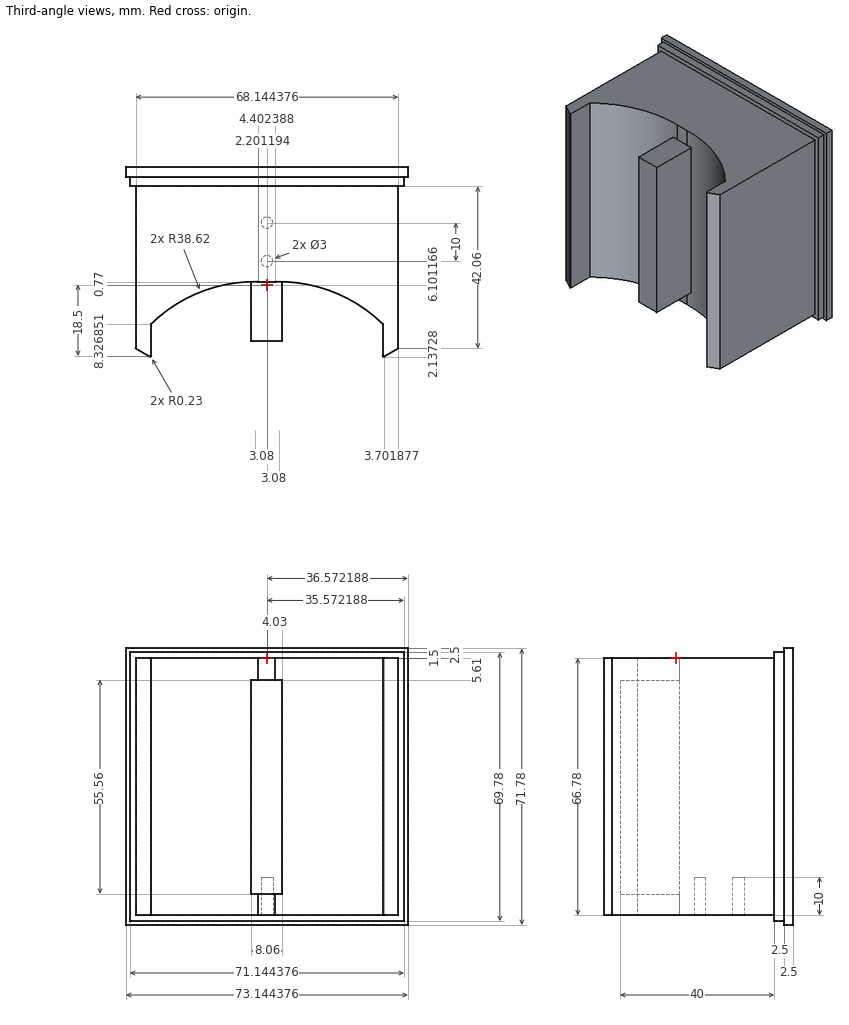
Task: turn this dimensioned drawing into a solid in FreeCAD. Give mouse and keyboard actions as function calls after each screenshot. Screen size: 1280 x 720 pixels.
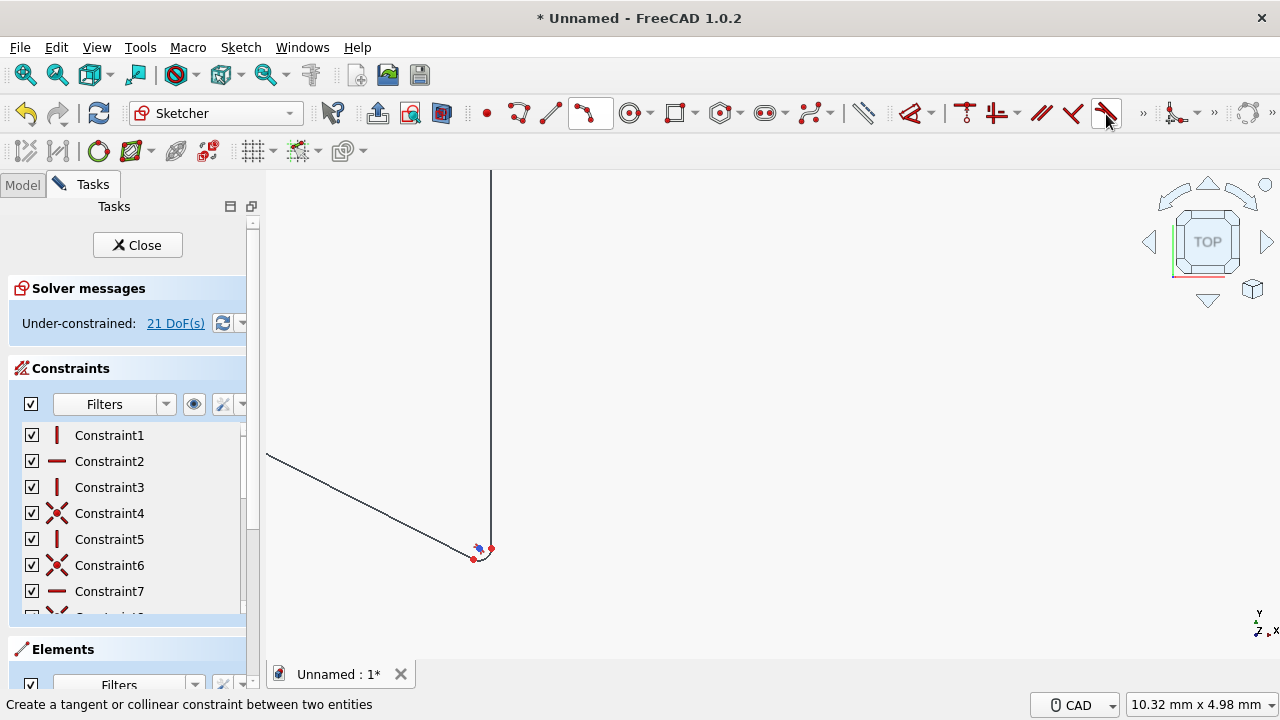
scroll(484, 577, down, 13)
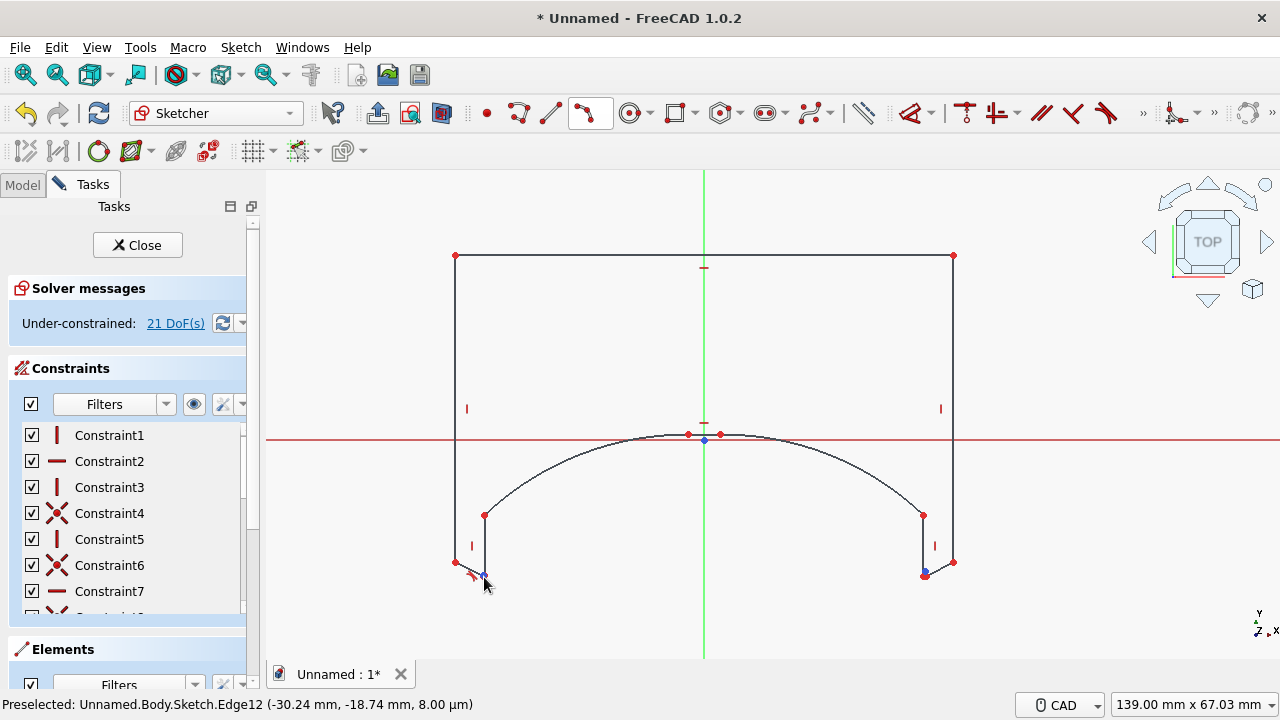
click(923, 534)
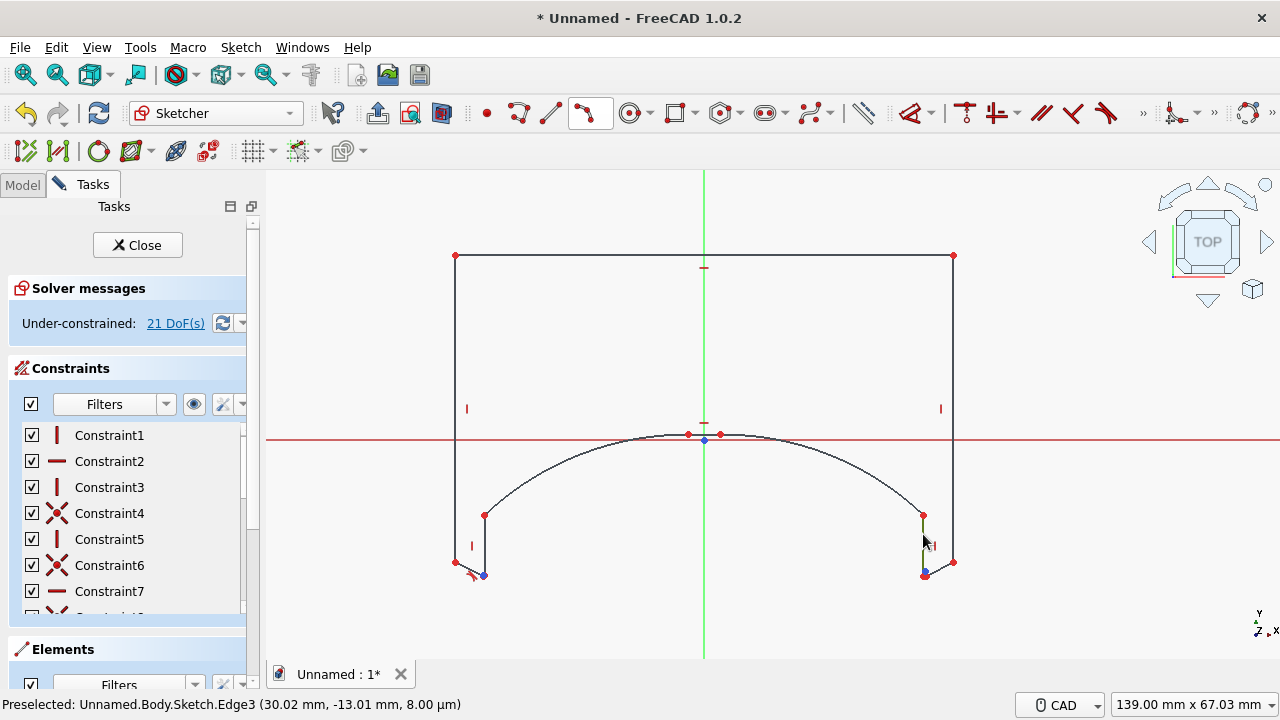
scroll(925, 577, up, 12)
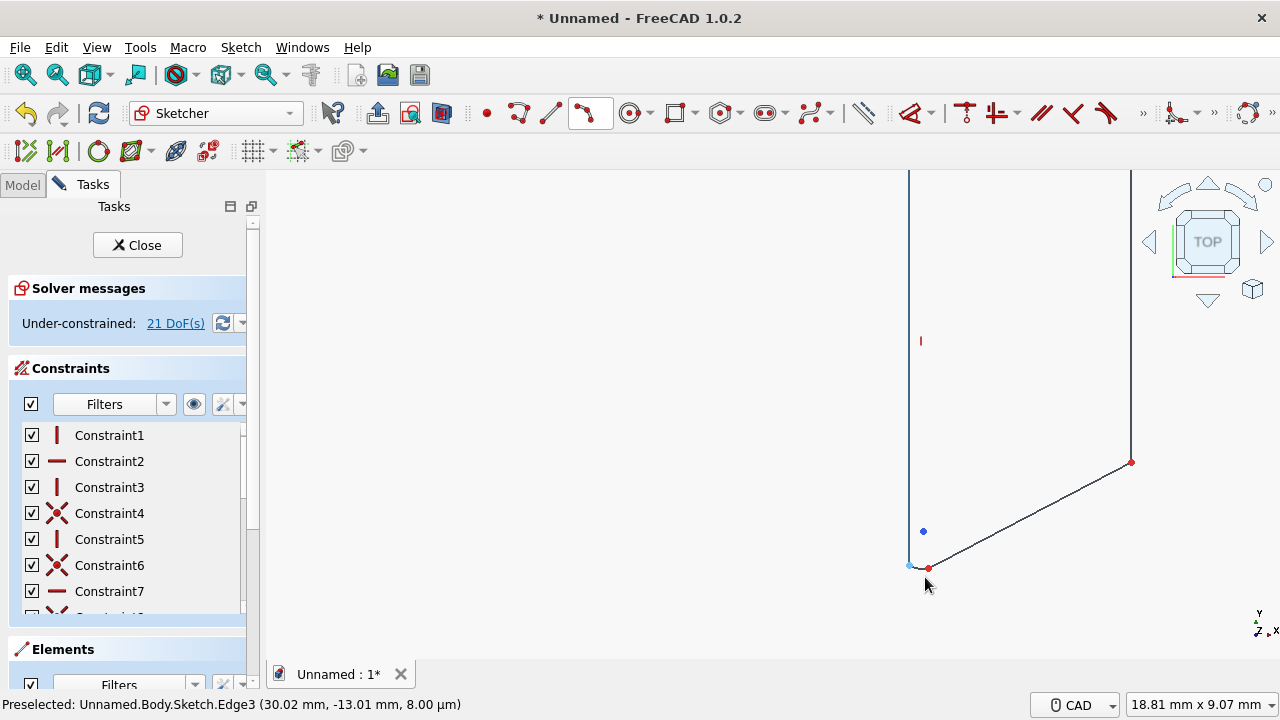
click(915, 564)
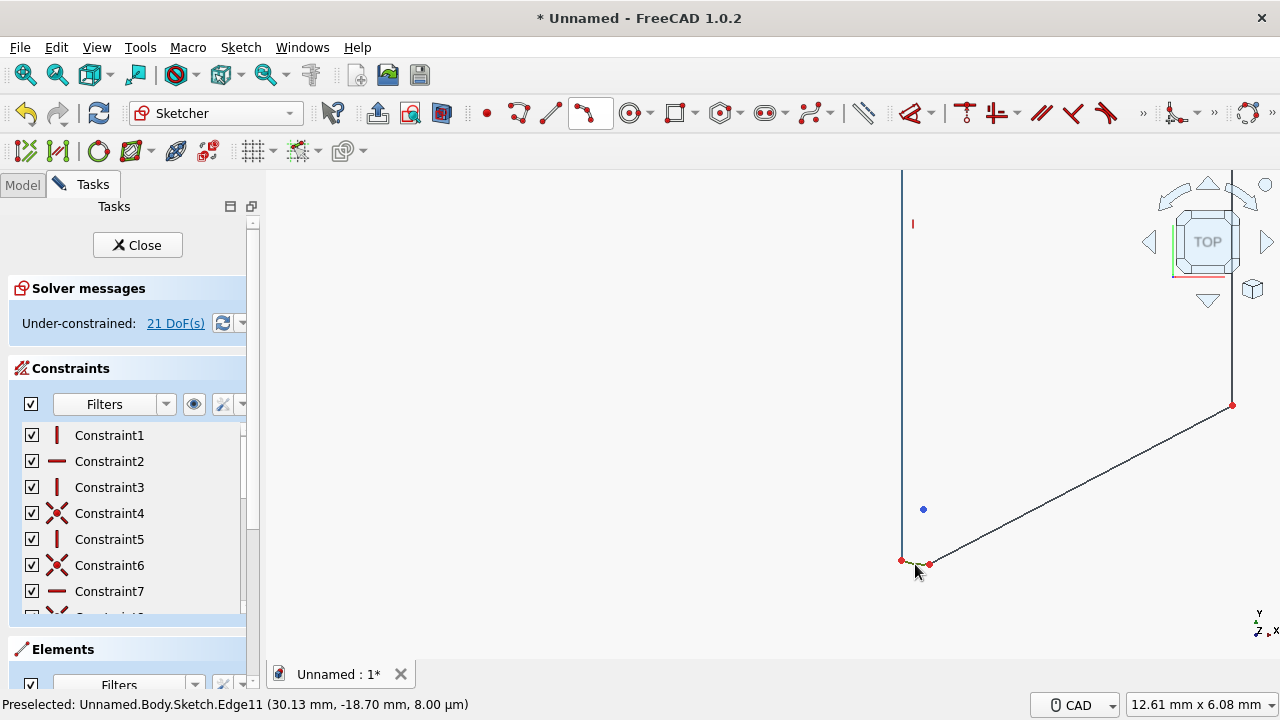
click(1106, 114)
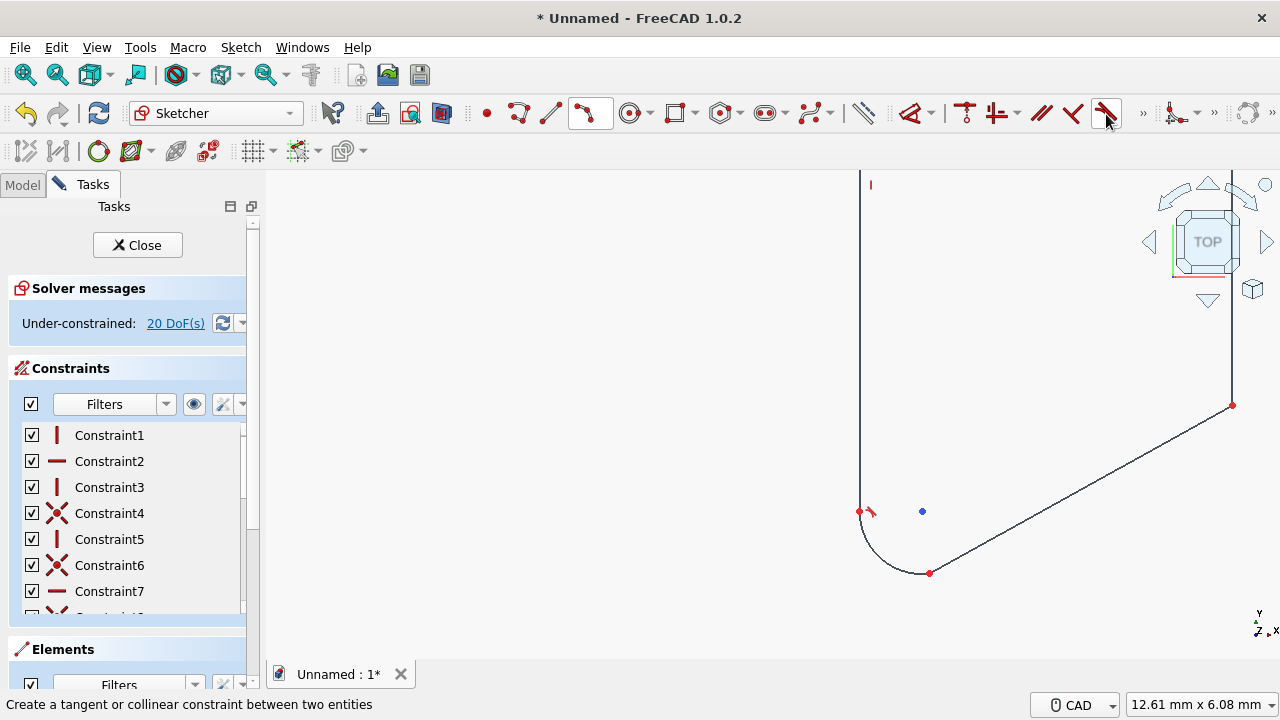
scroll(926, 577, down, 12)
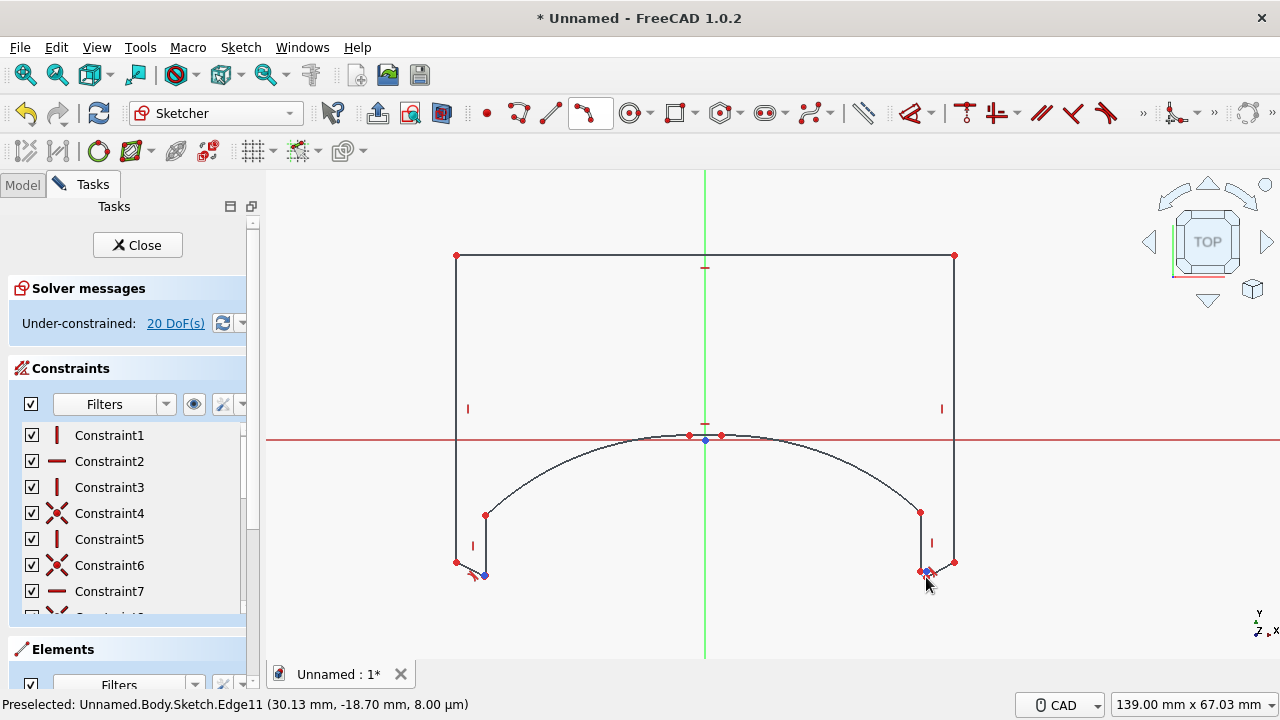
scroll(935, 573, up, 2)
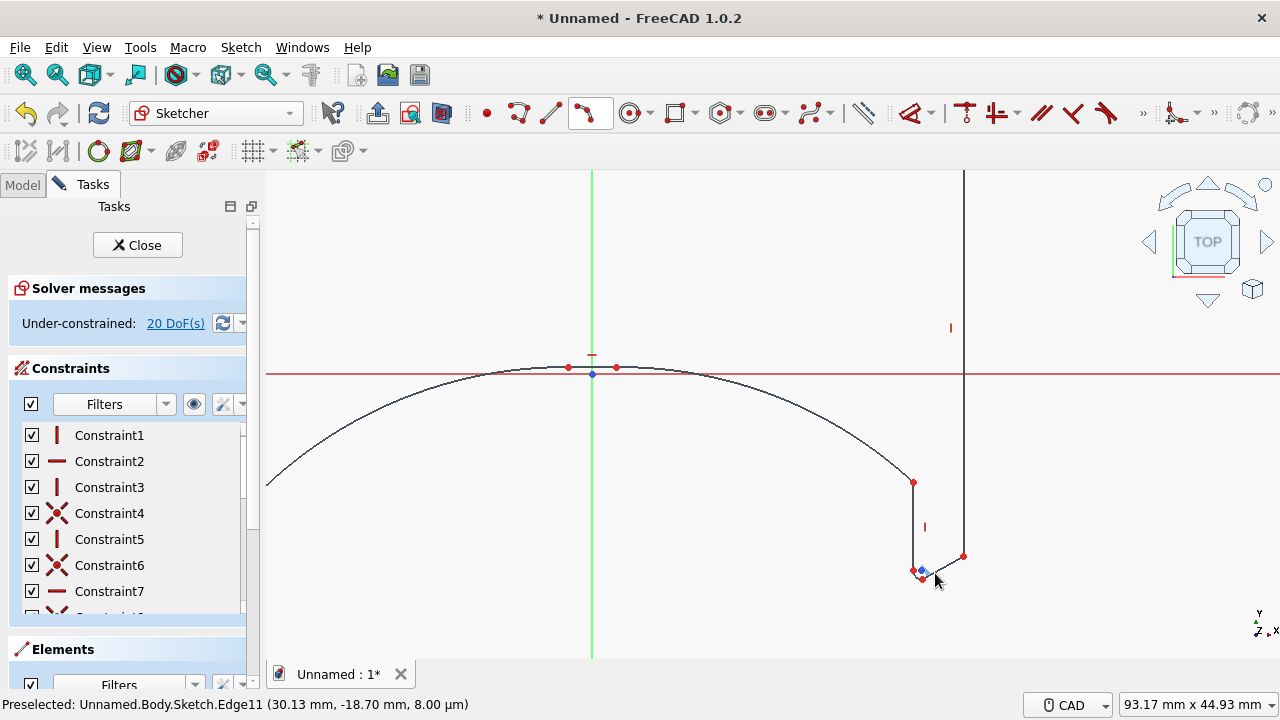
click(935, 572)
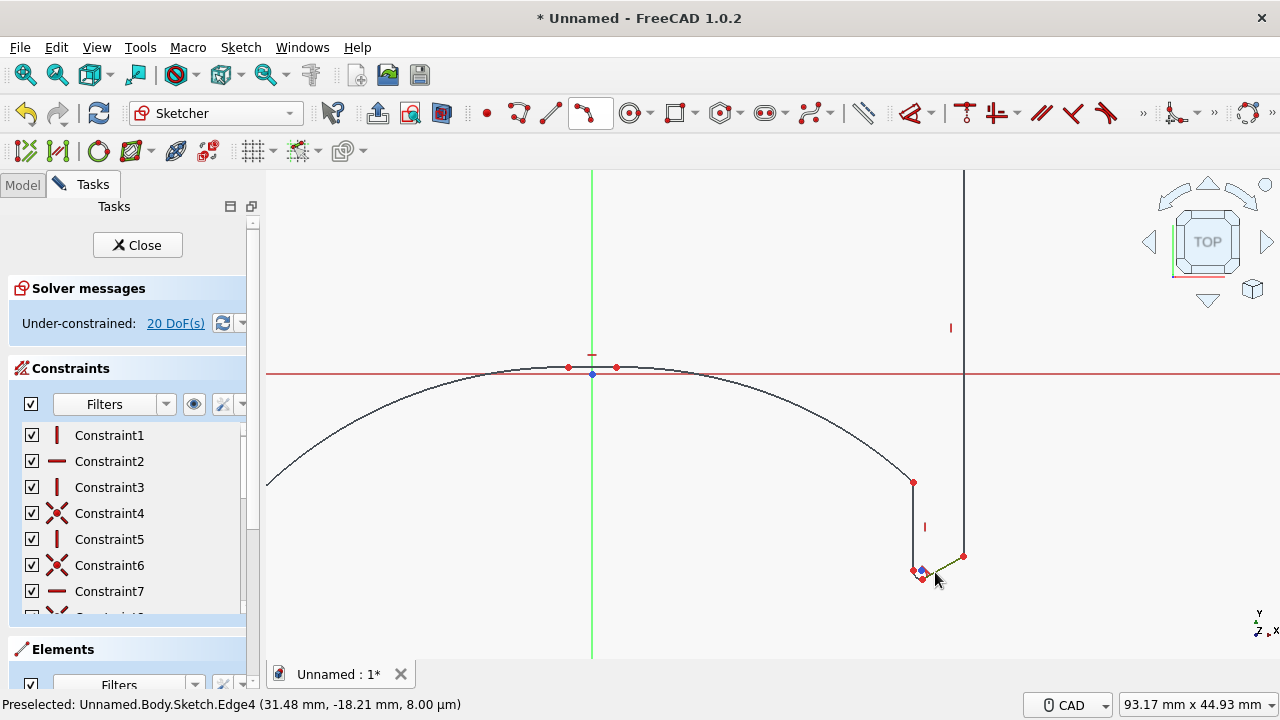
scroll(916, 577, up, 4)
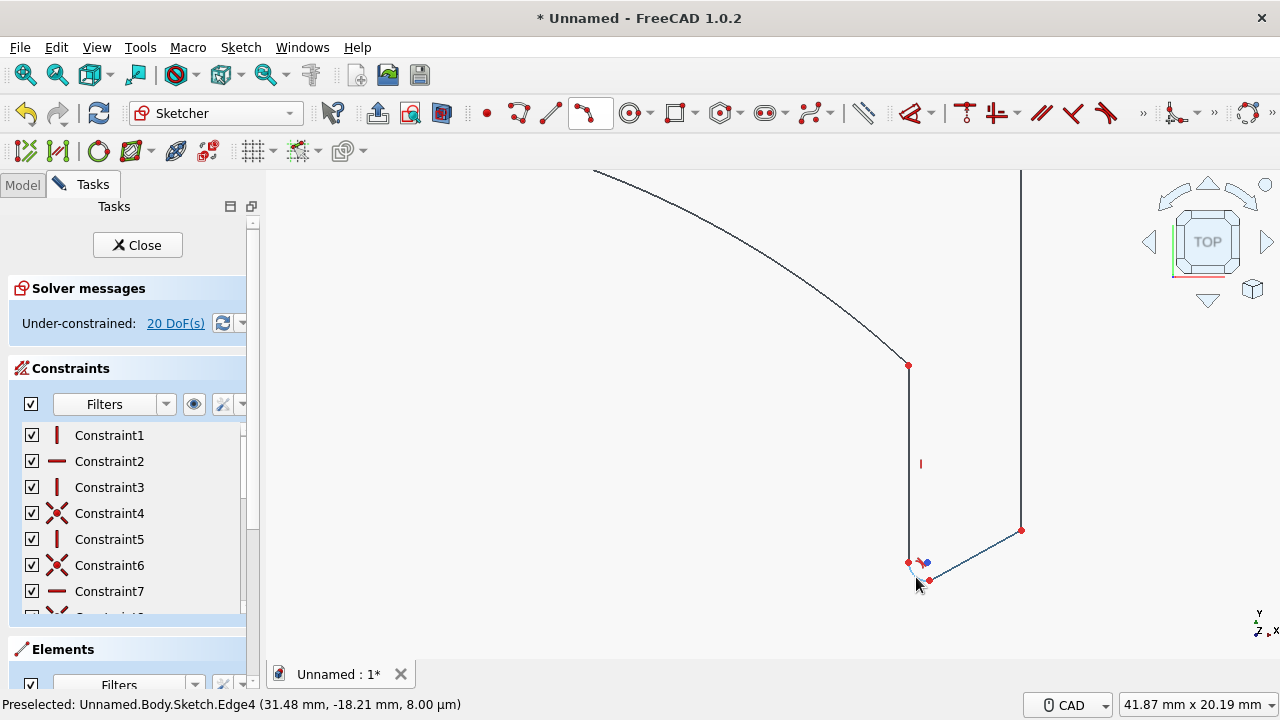
click(915, 576)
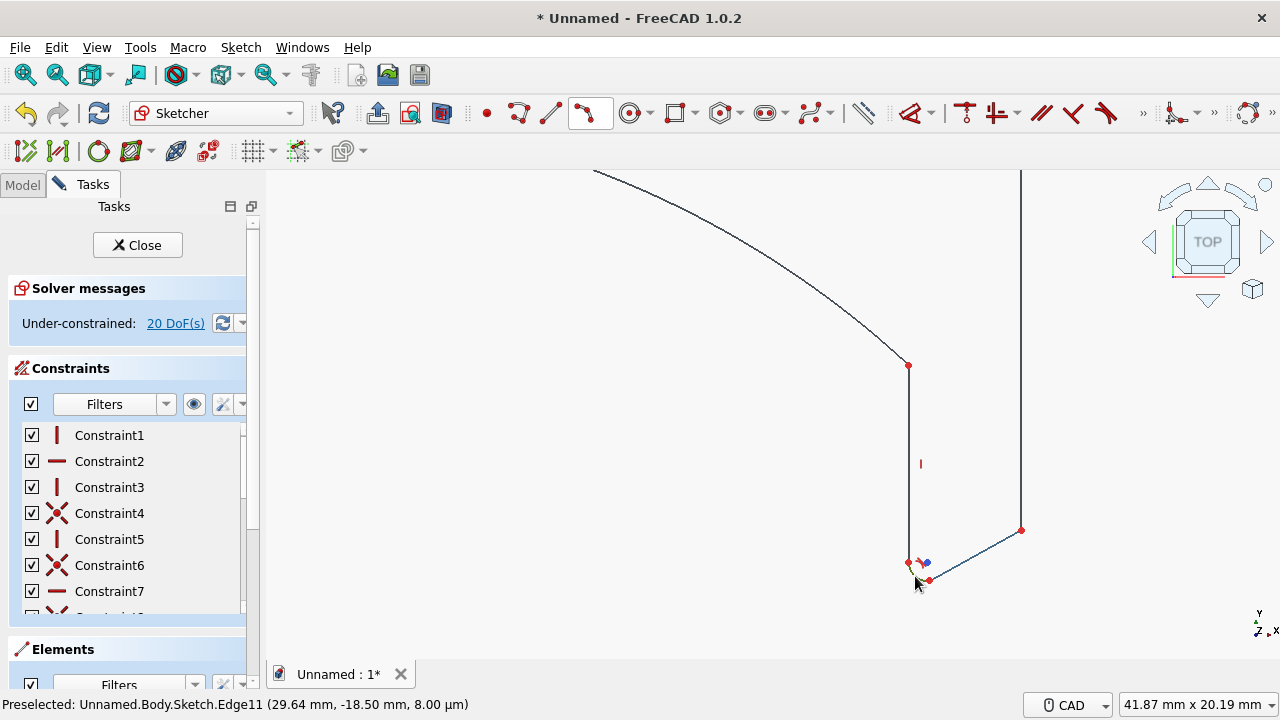
click(1106, 114)